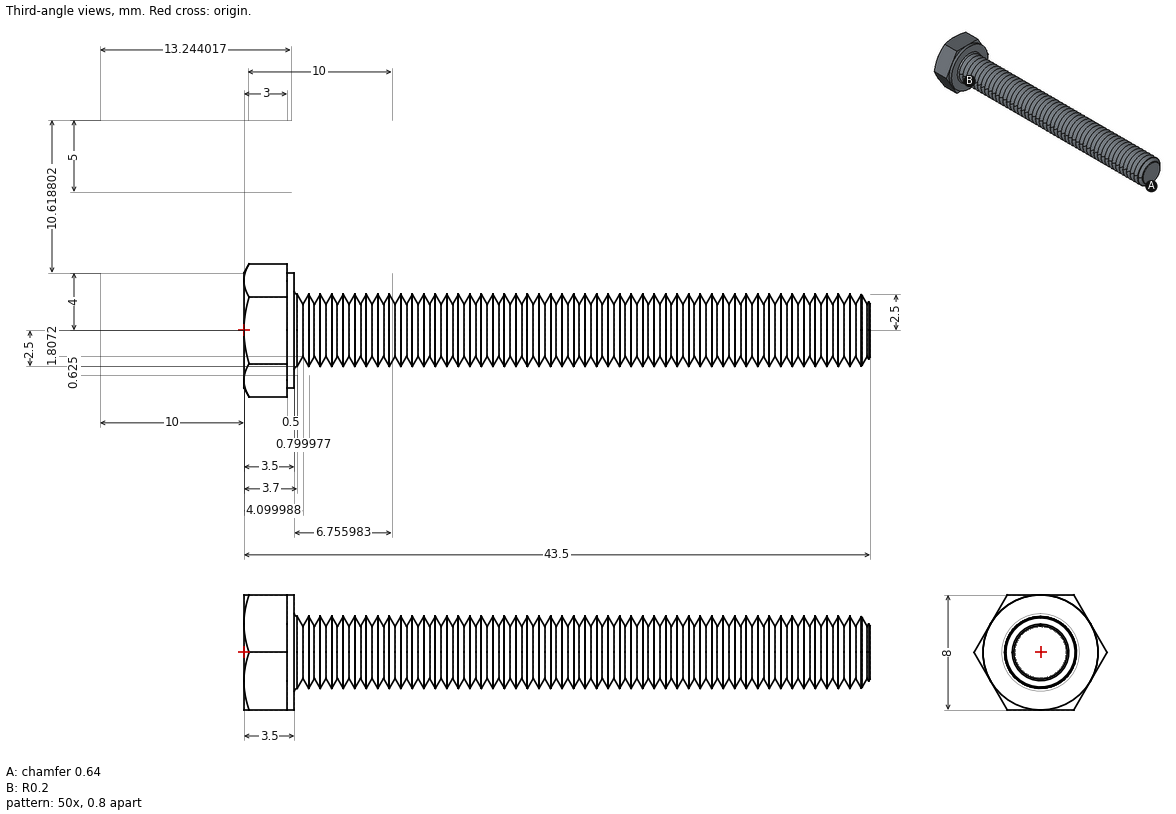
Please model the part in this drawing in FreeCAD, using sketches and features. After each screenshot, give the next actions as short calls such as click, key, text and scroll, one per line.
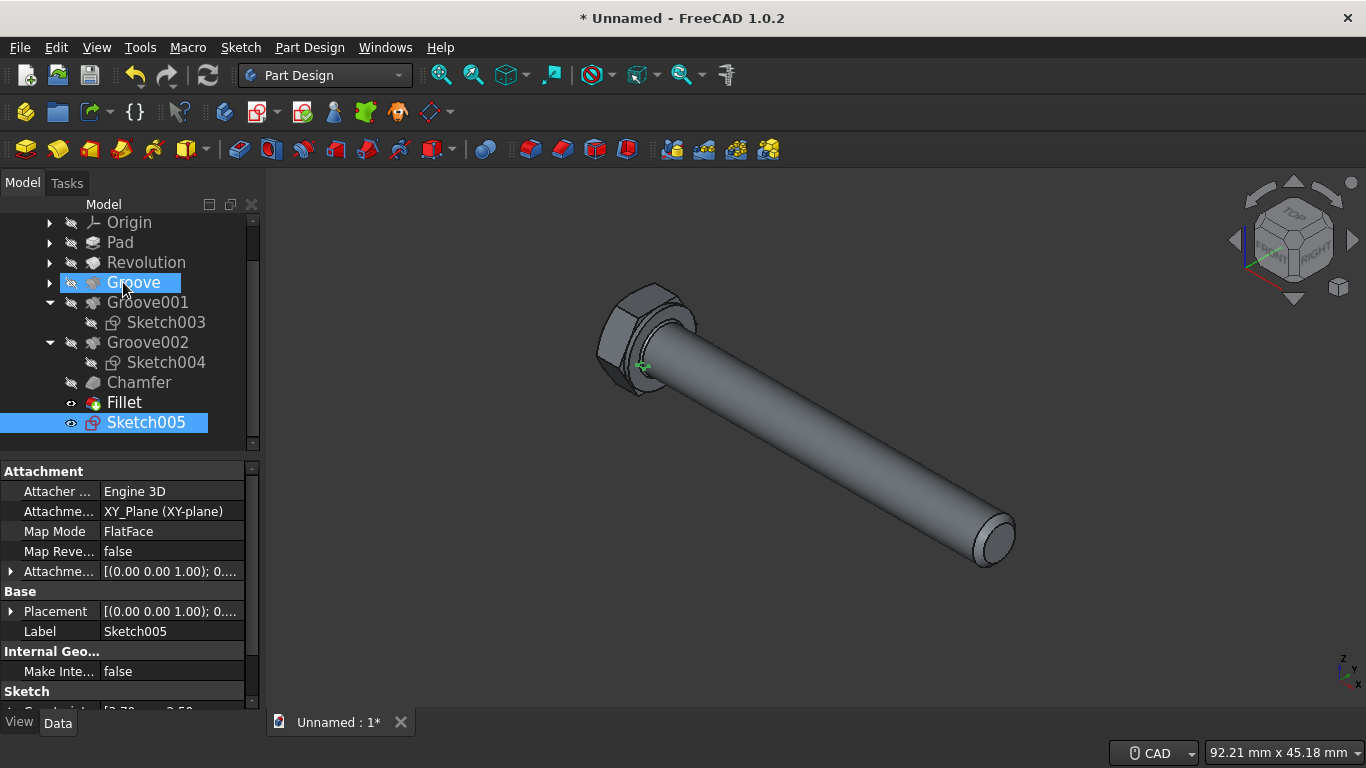
click(304, 150)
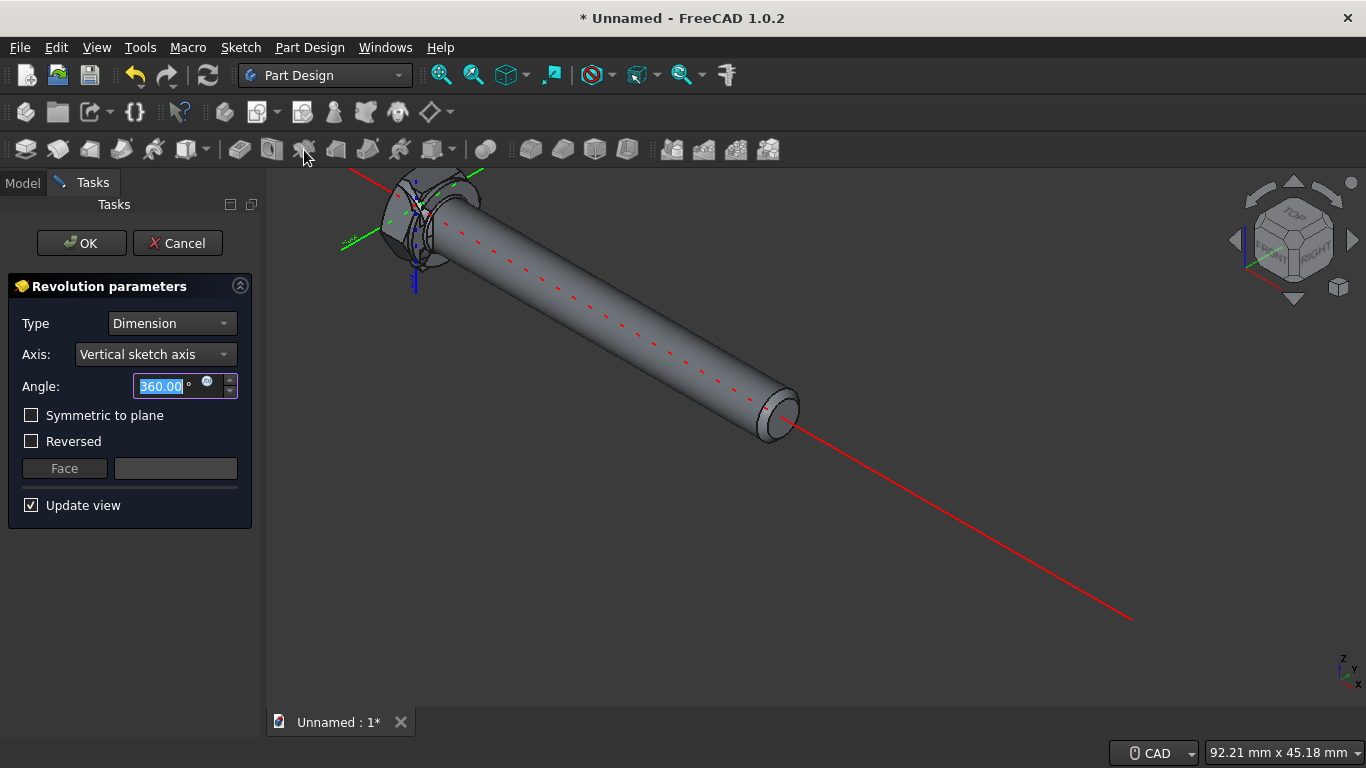
click(156, 354)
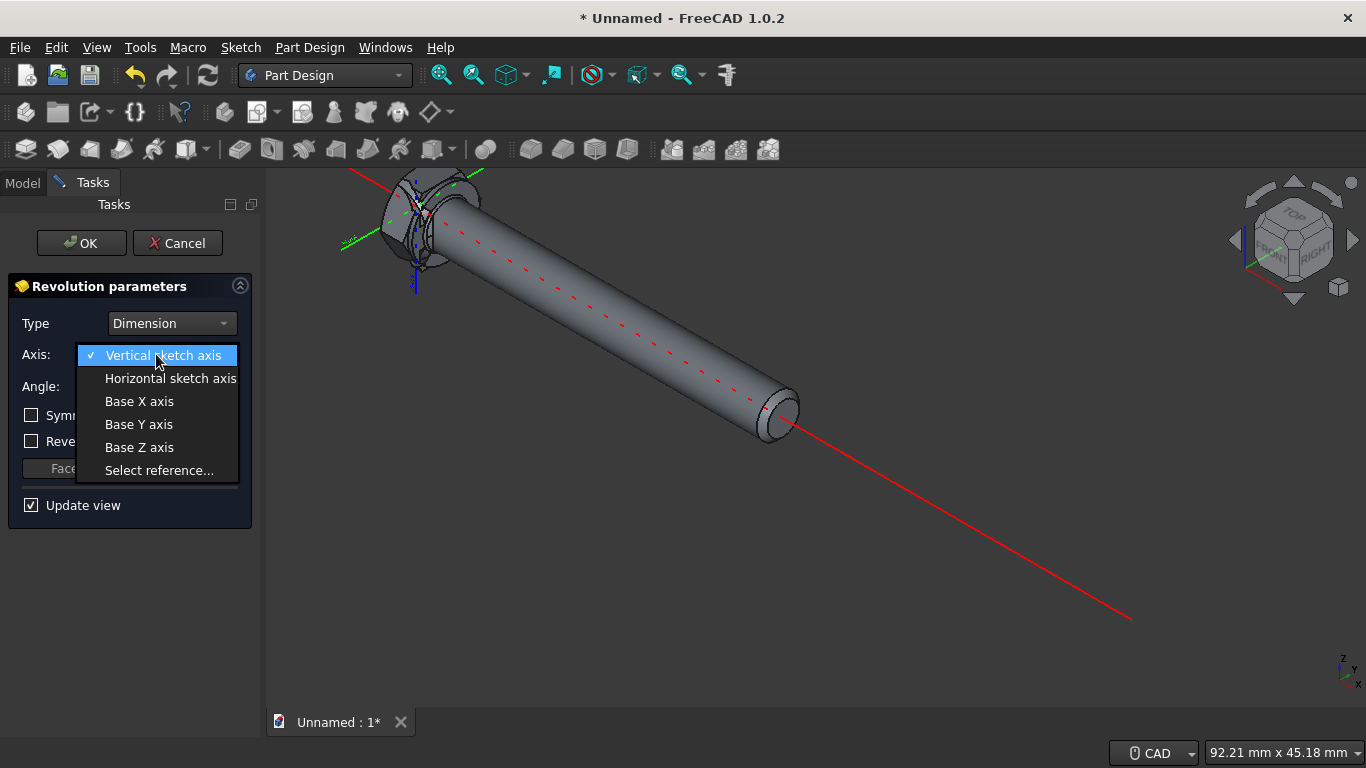
click(156, 378)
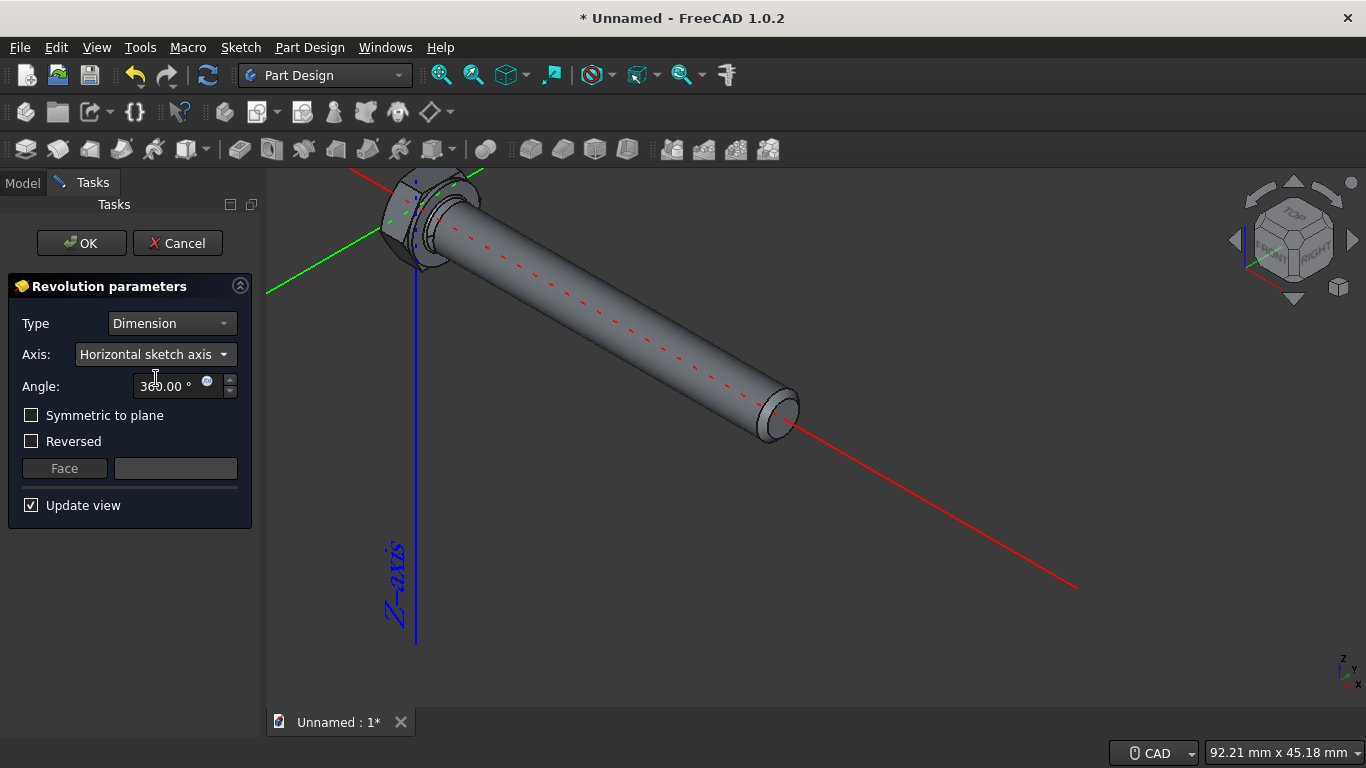
click(82, 243)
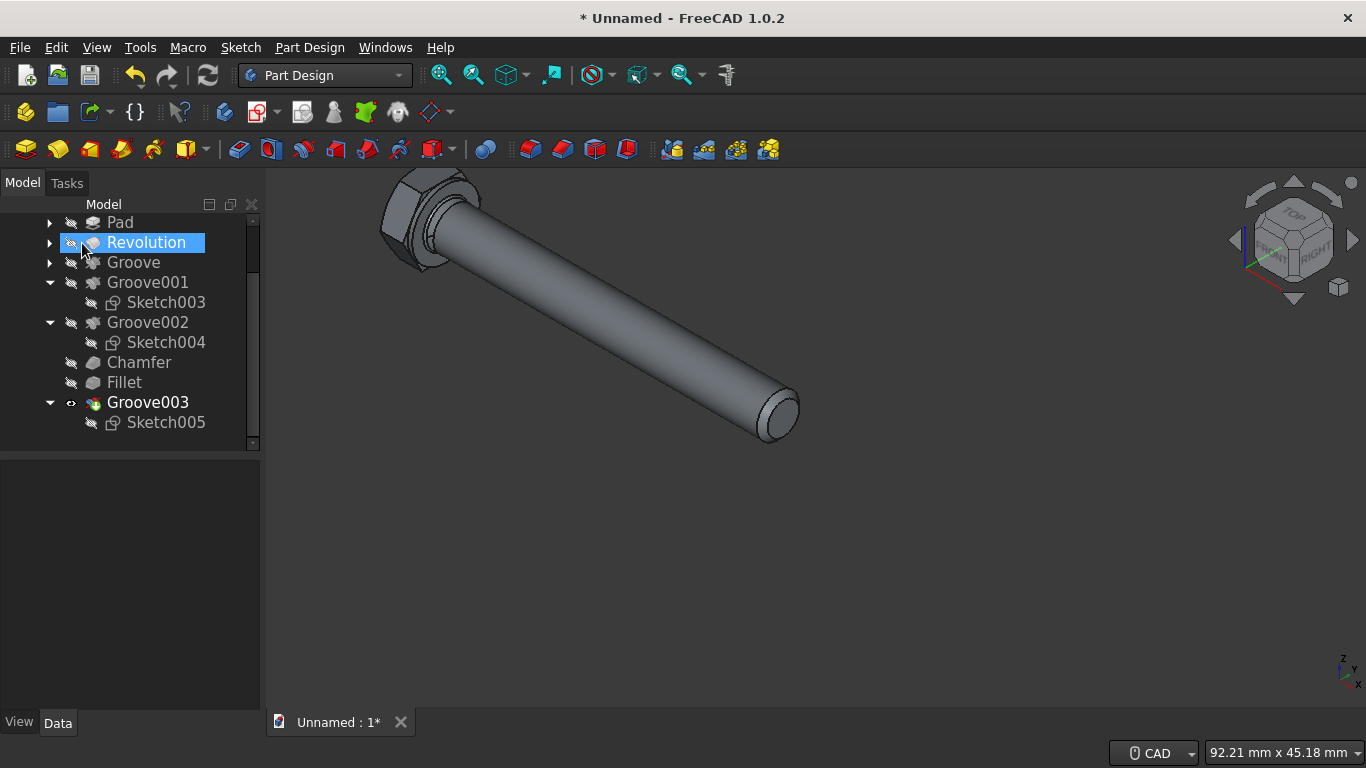
click(442, 76)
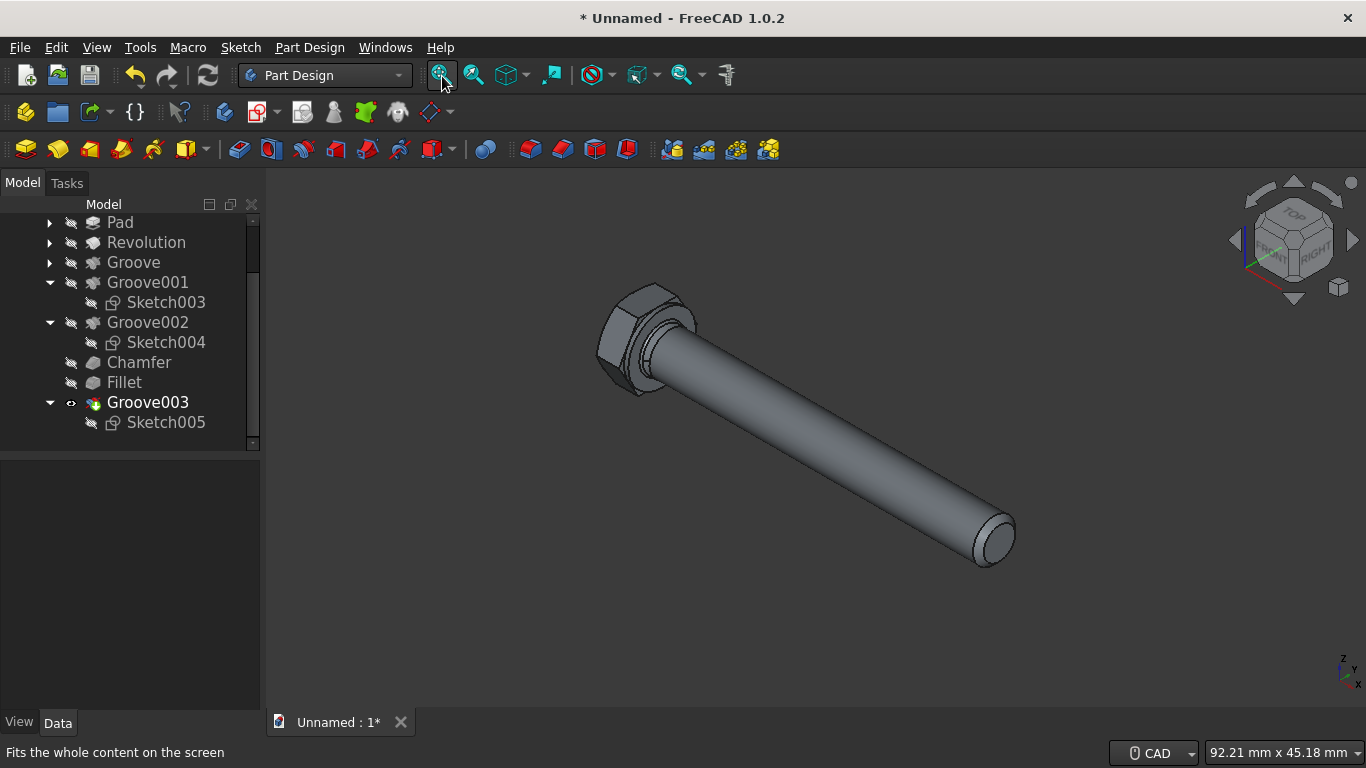
click(116, 403)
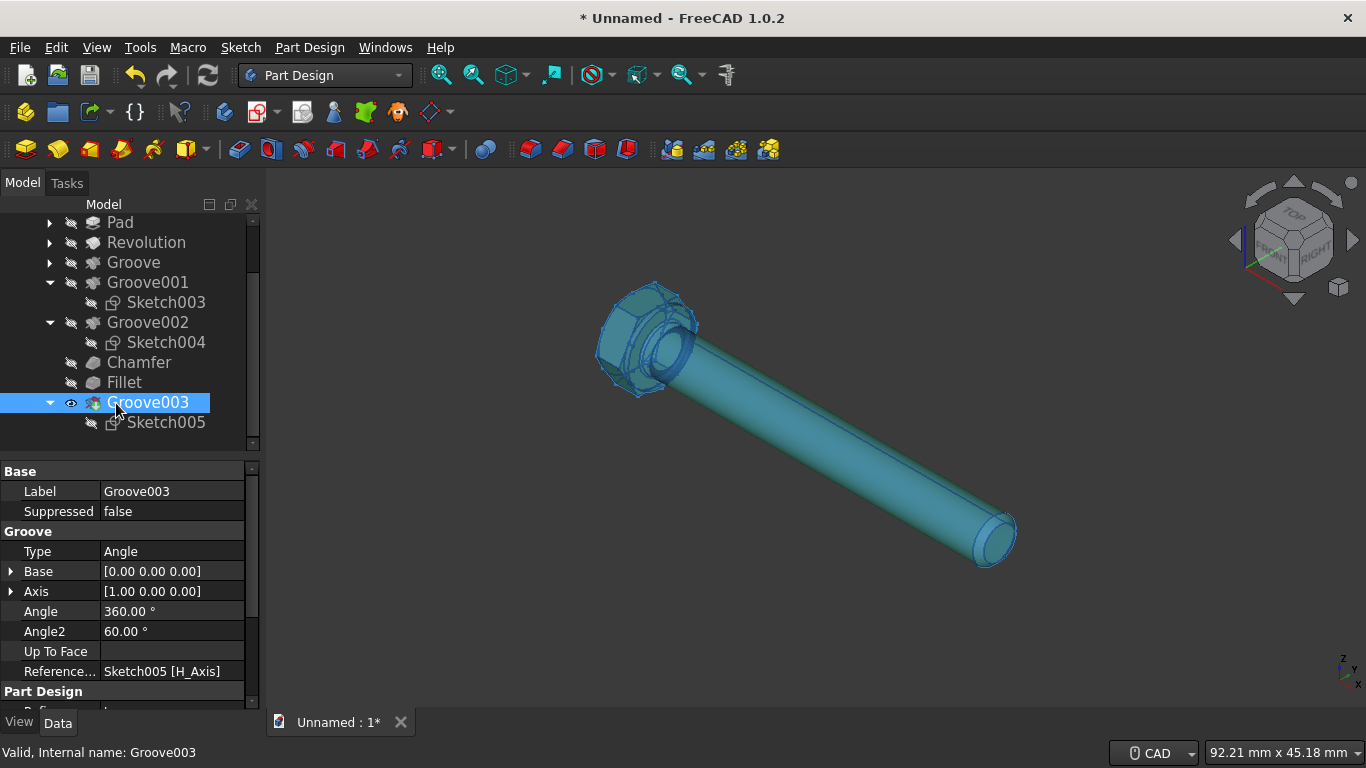
click(704, 150)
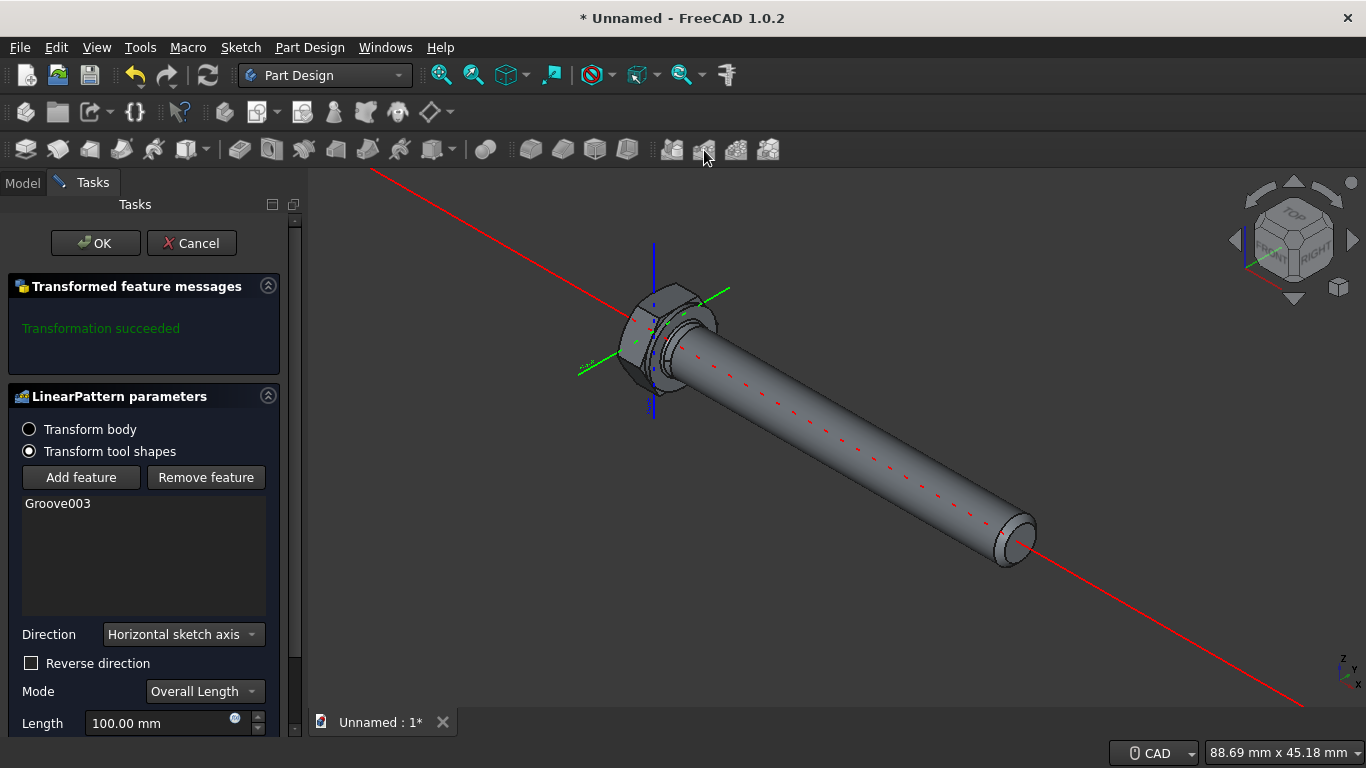
click(184, 634)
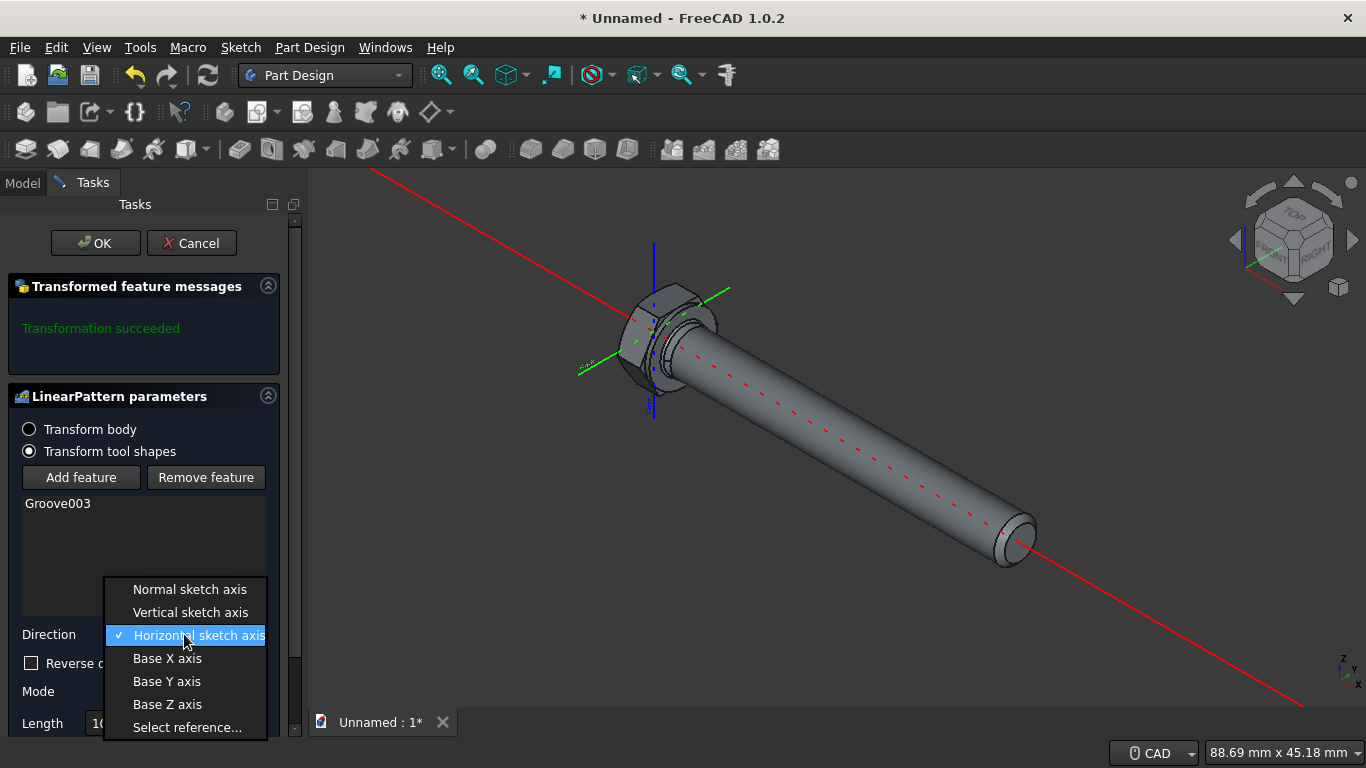
click(184, 658)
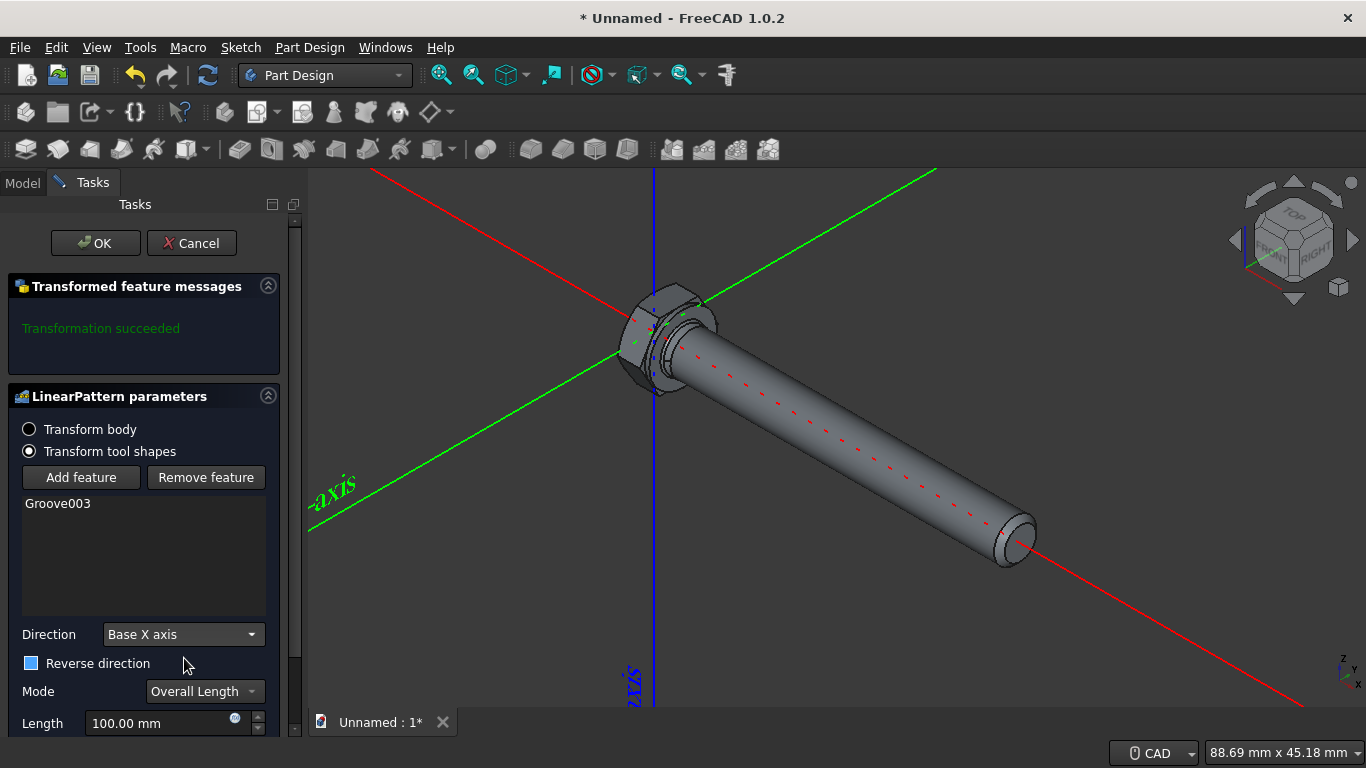
click(206, 692)